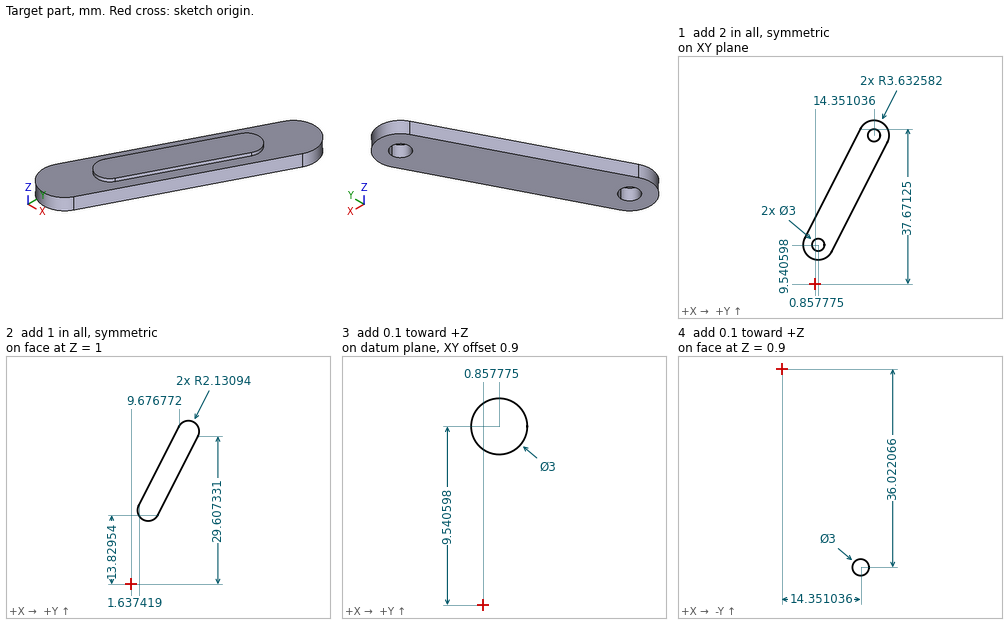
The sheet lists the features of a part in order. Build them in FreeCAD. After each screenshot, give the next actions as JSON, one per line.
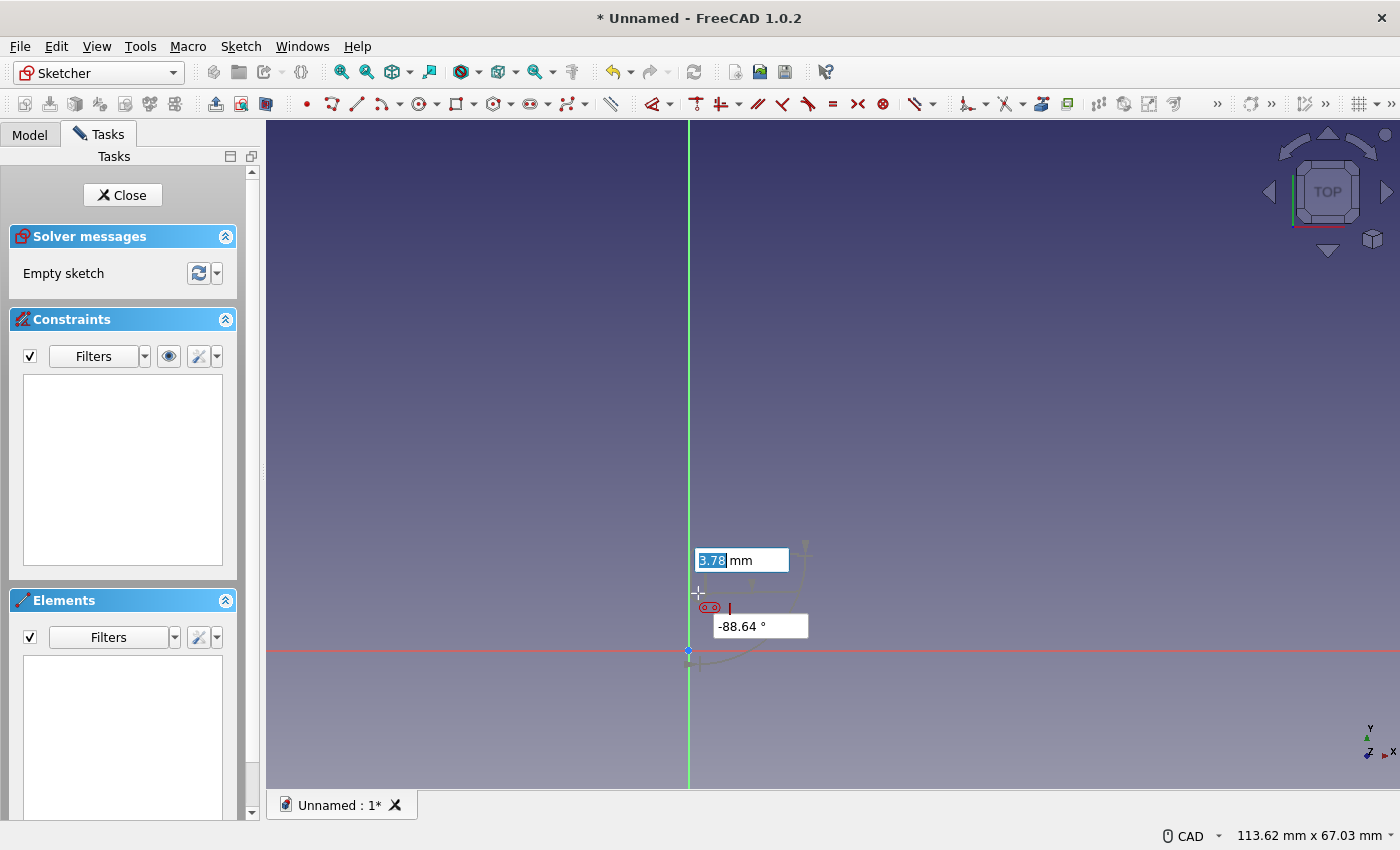
{"action": "left_click", "coordinate": [832, 291]}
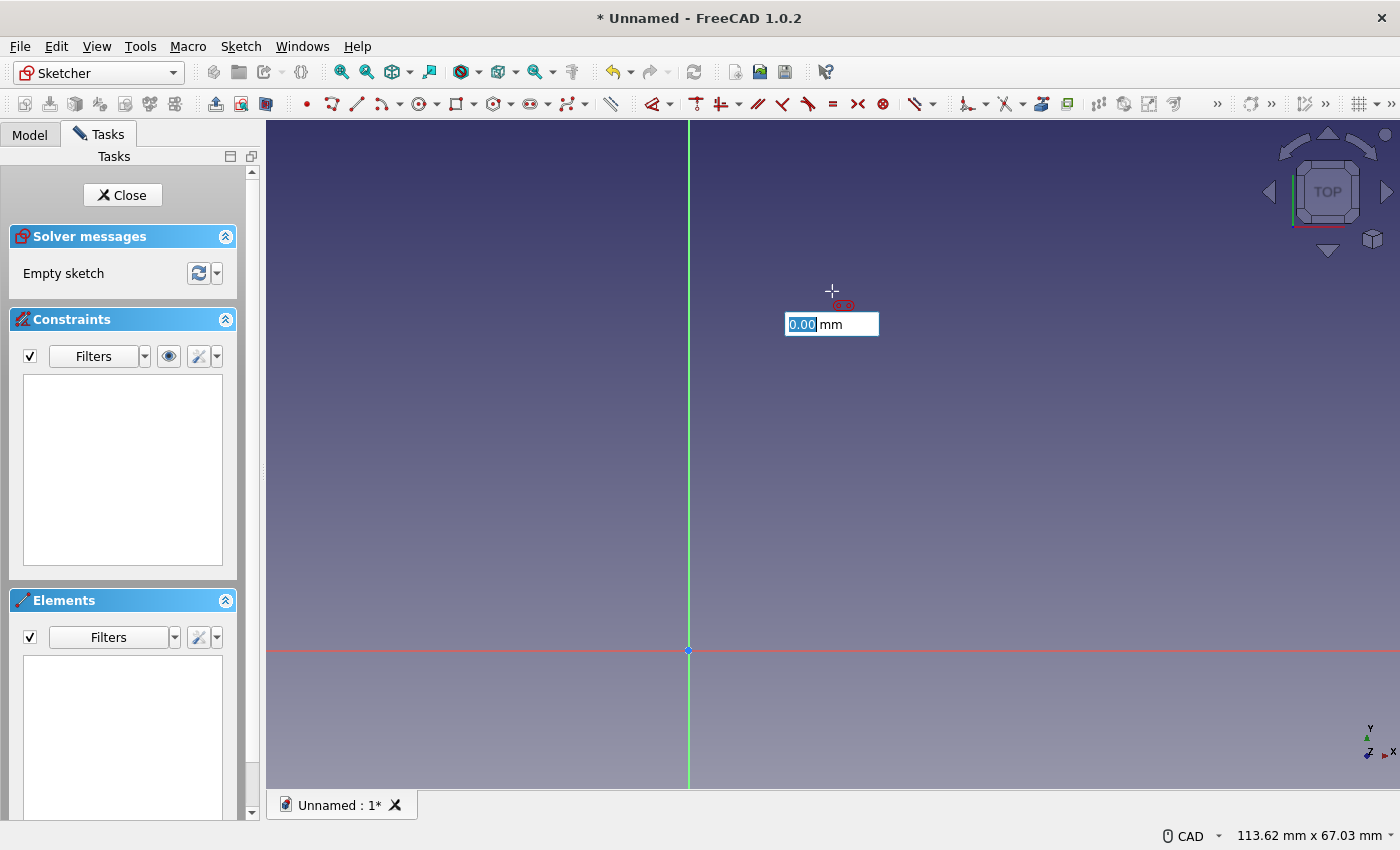
{"action": "left_click", "coordinate": [732, 407]}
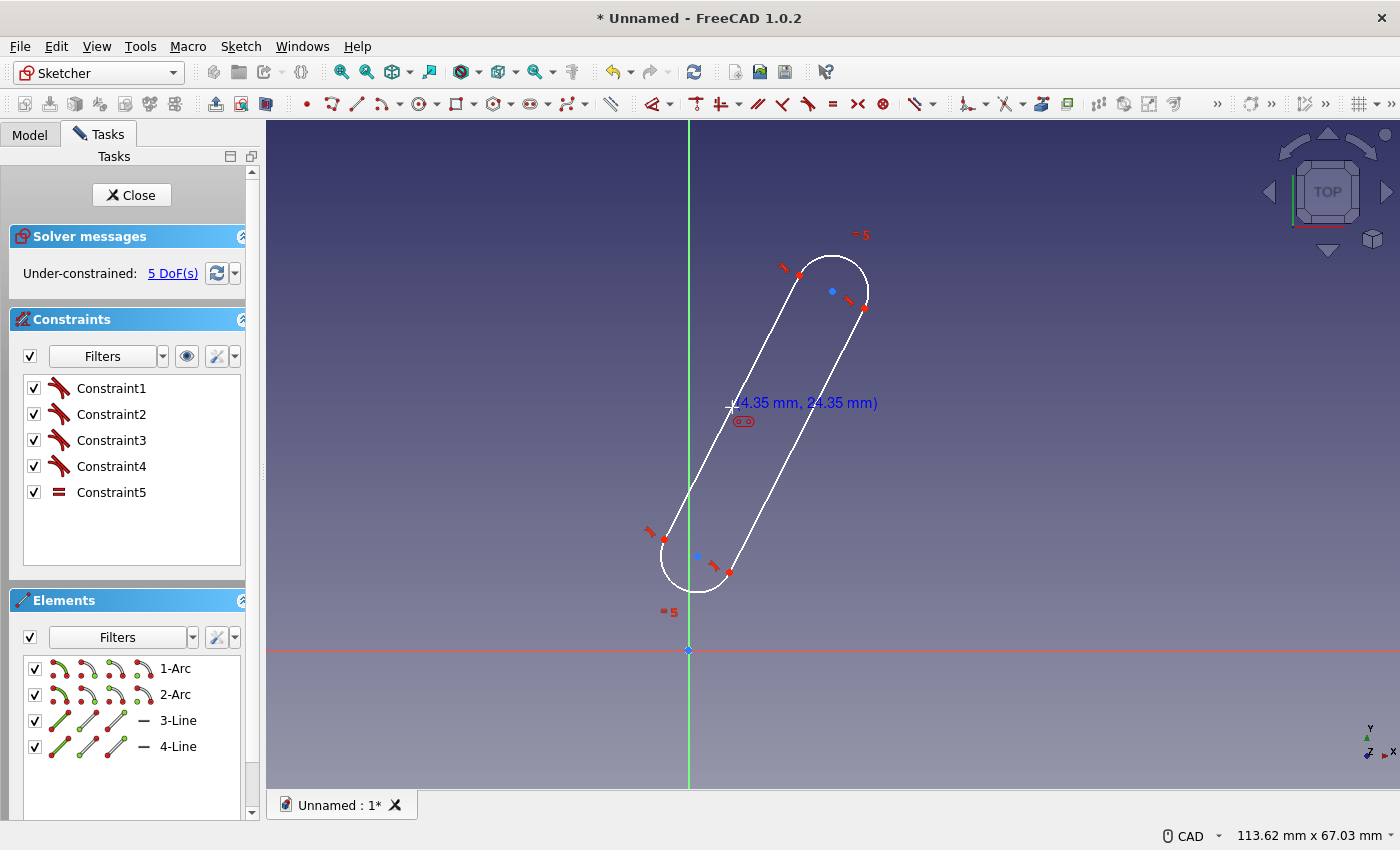
{"action": "key", "text": "g c"}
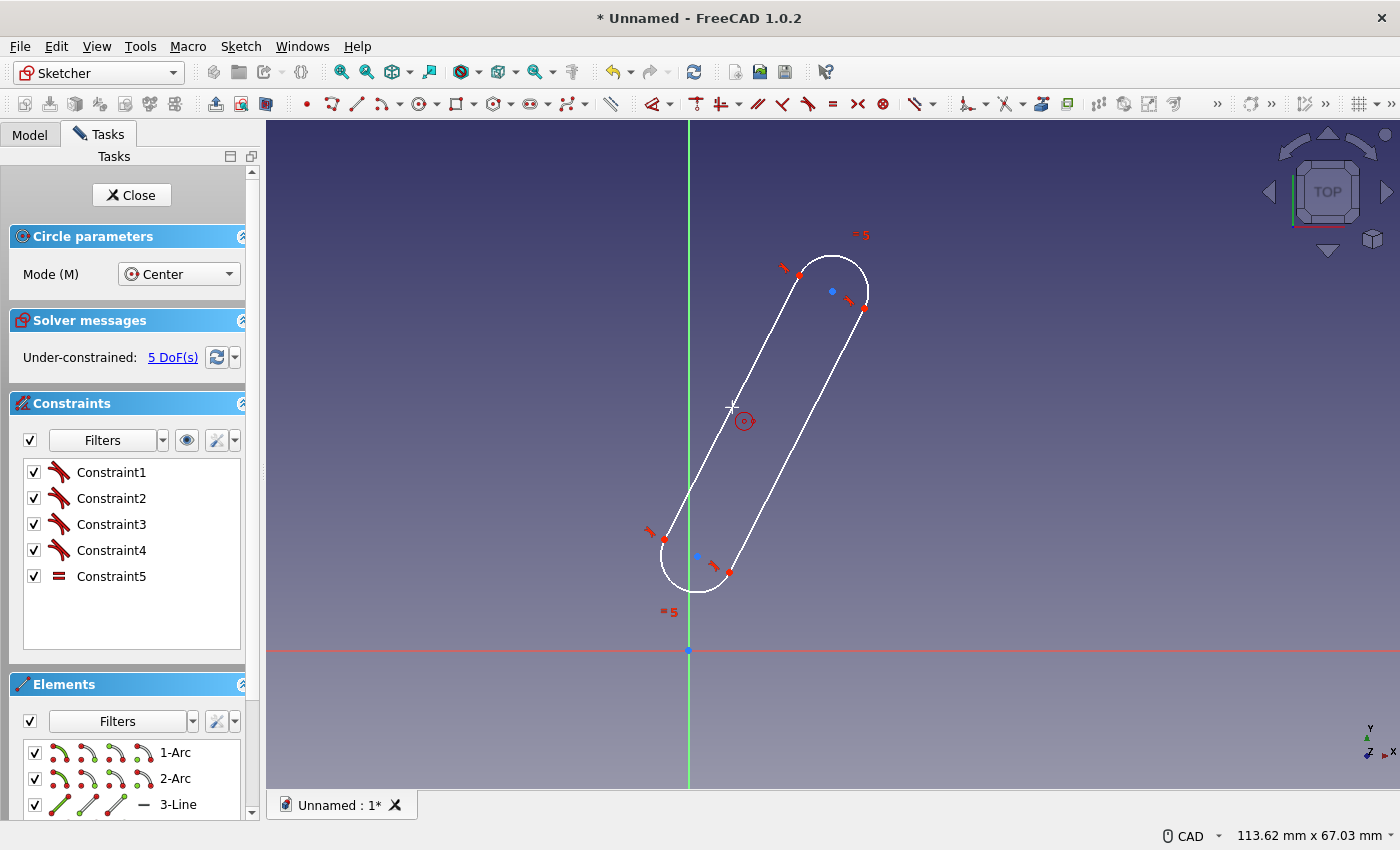
{"action": "scroll", "coordinate": [697, 556], "scroll_direction": "up", "scroll_amount": 4}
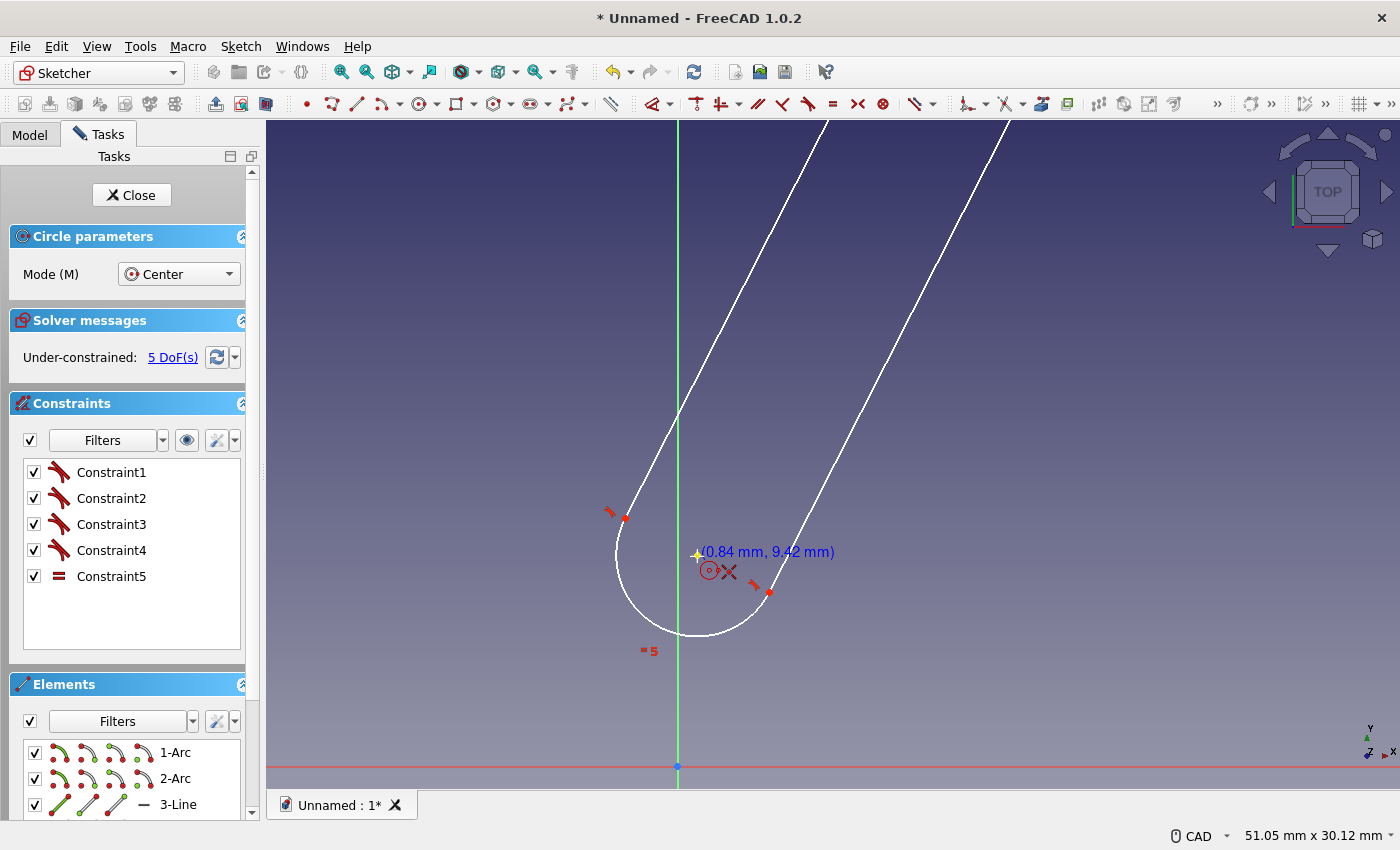
{"action": "left_click", "coordinate": [697, 555]}
{"action": "left_click", "coordinate": [720, 531]}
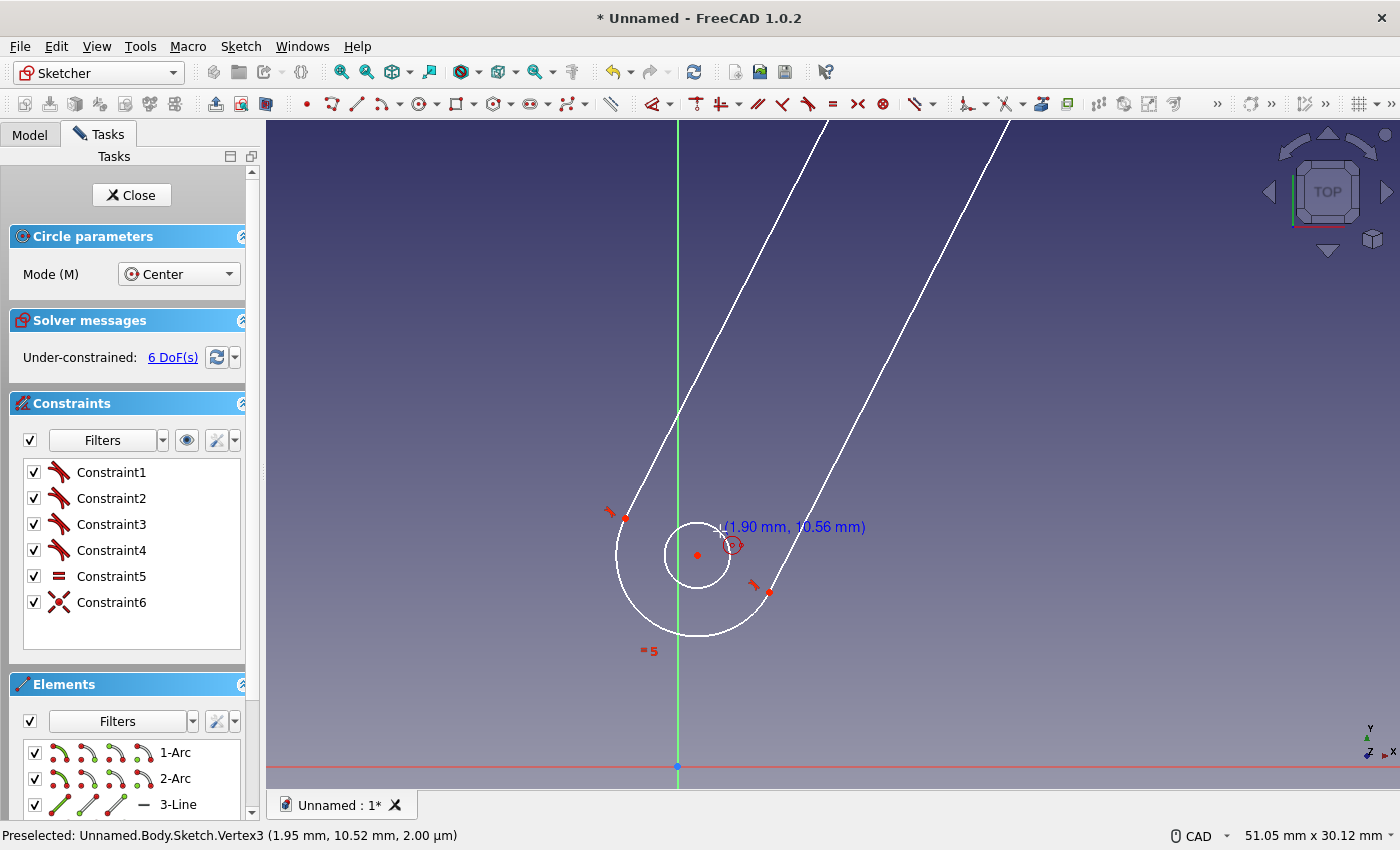
{"action": "scroll", "coordinate": [697, 556], "scroll_direction": "down", "scroll_amount": 4}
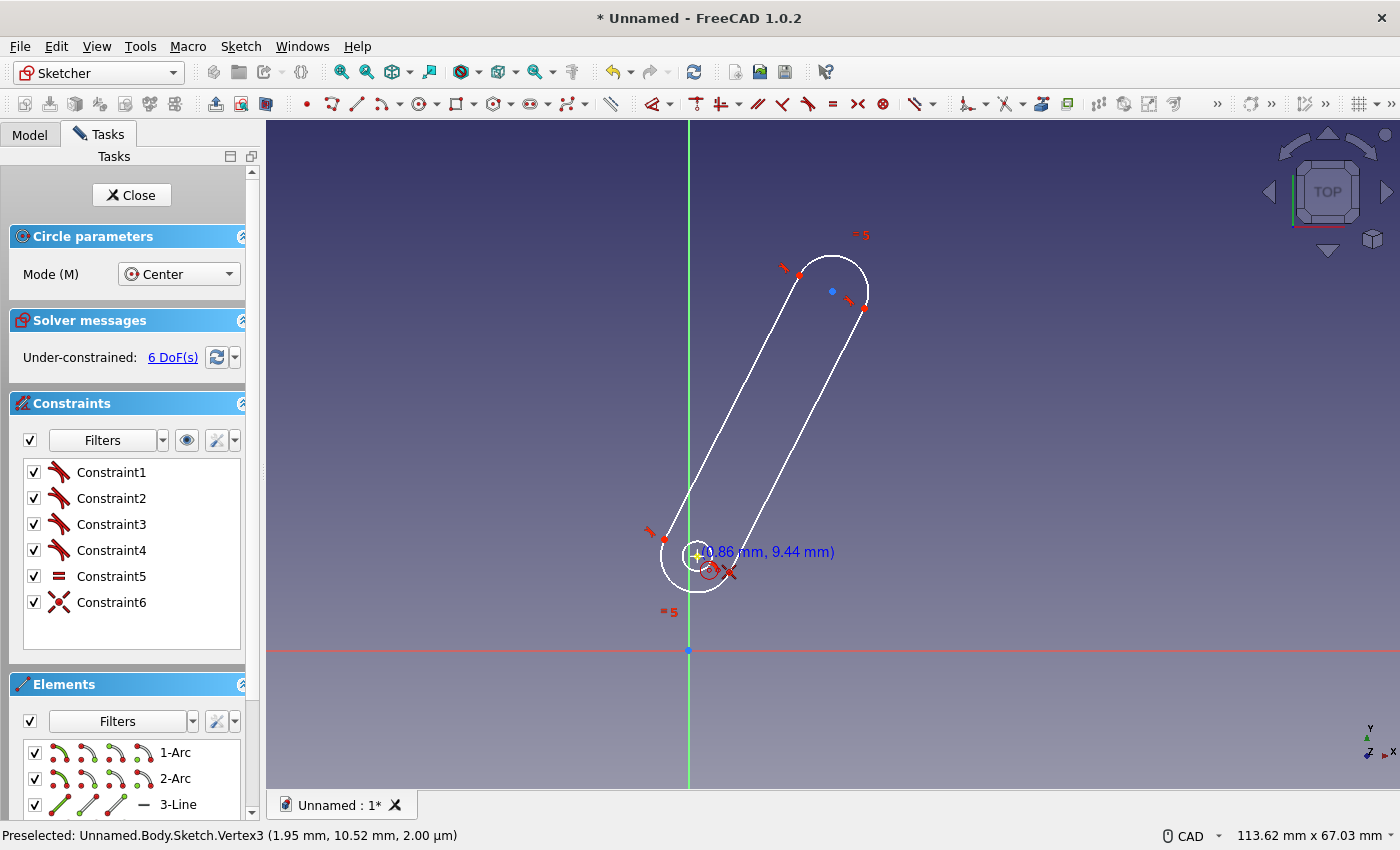
{"action": "scroll", "coordinate": [832, 291], "scroll_direction": "up", "scroll_amount": 3}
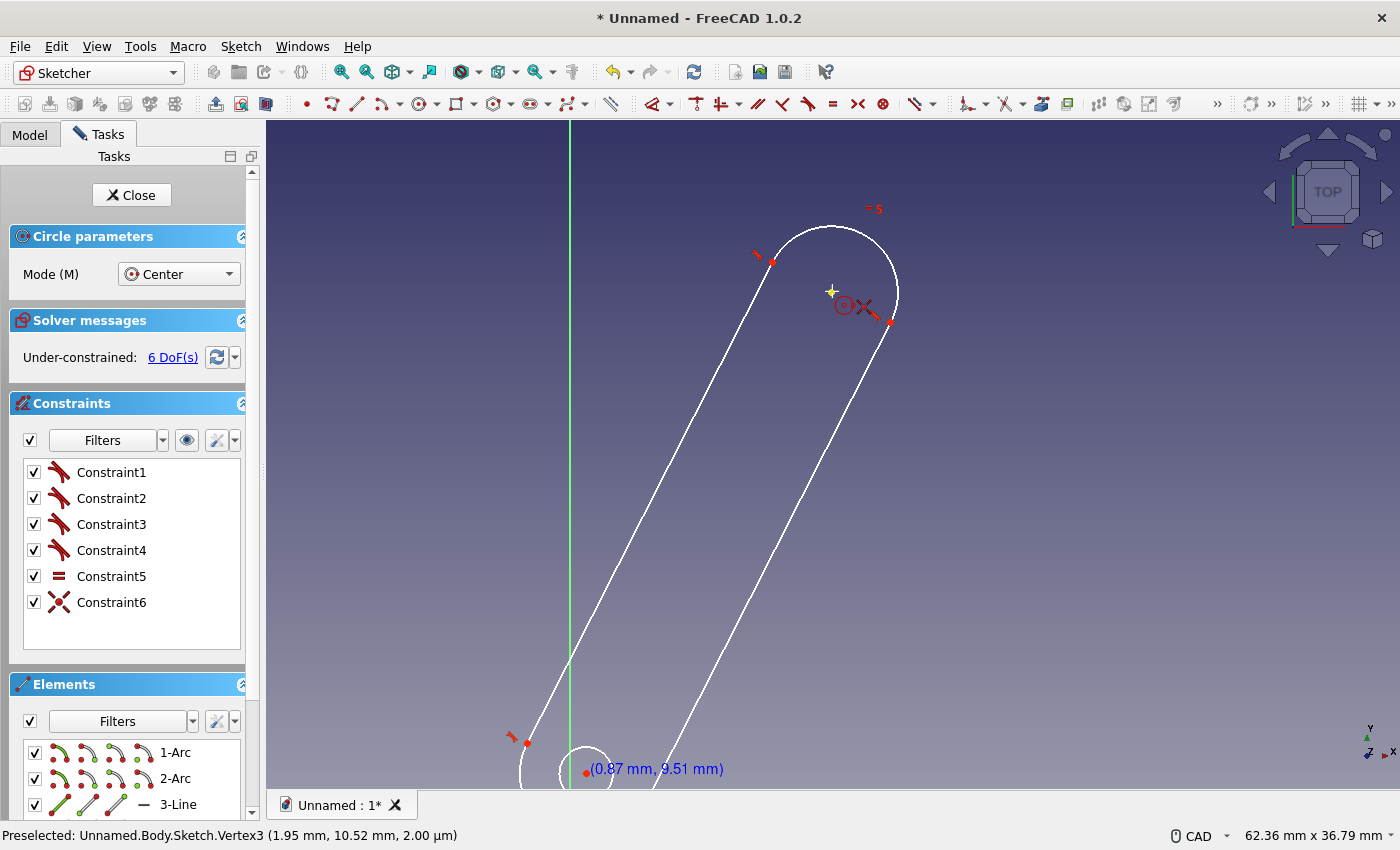
{"action": "left_click", "coordinate": [832, 293]}
{"action": "left_click", "coordinate": [851, 272]}
{"action": "key", "text": "Escape"}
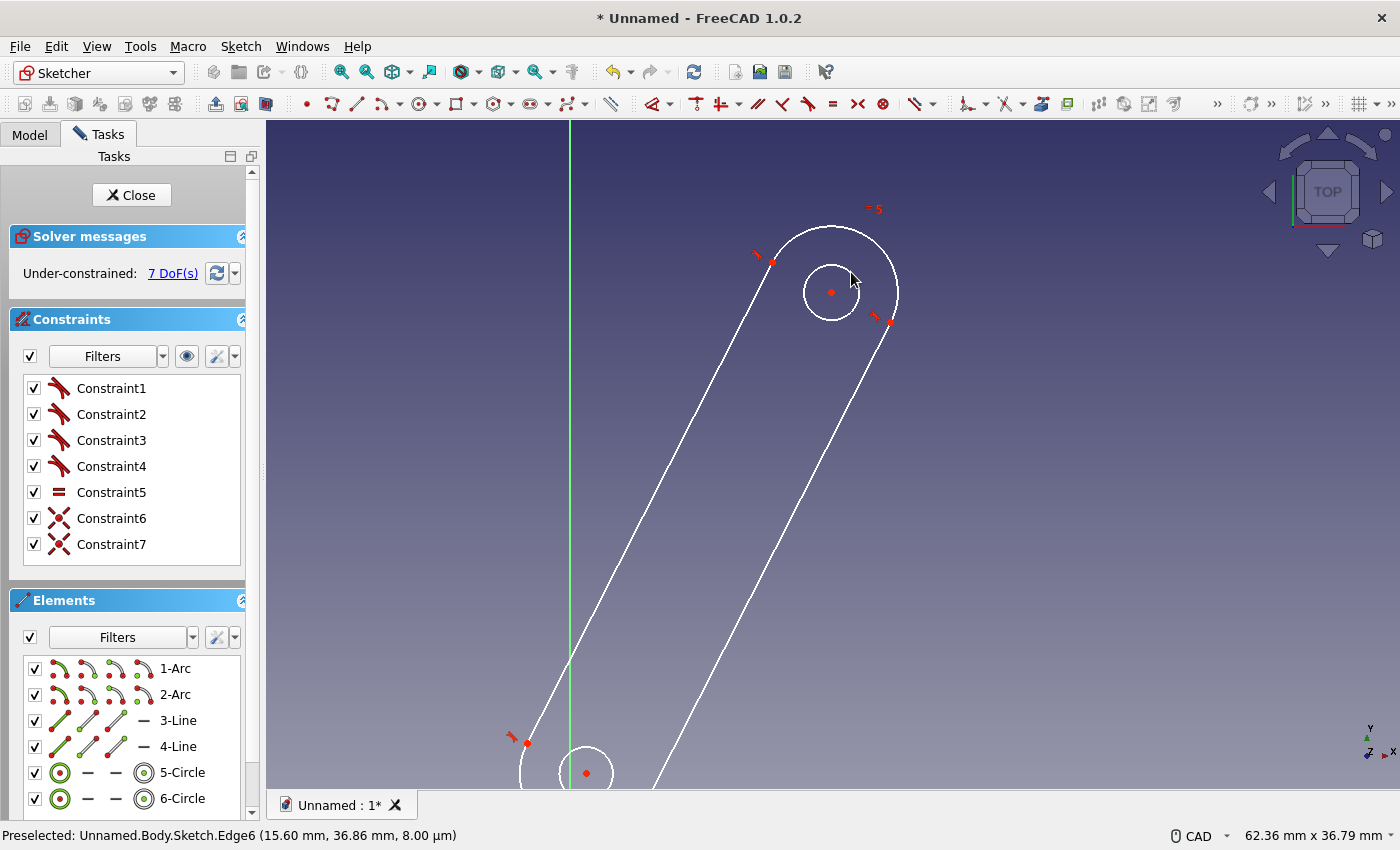
{"action": "left_click", "coordinate": [605, 755]}